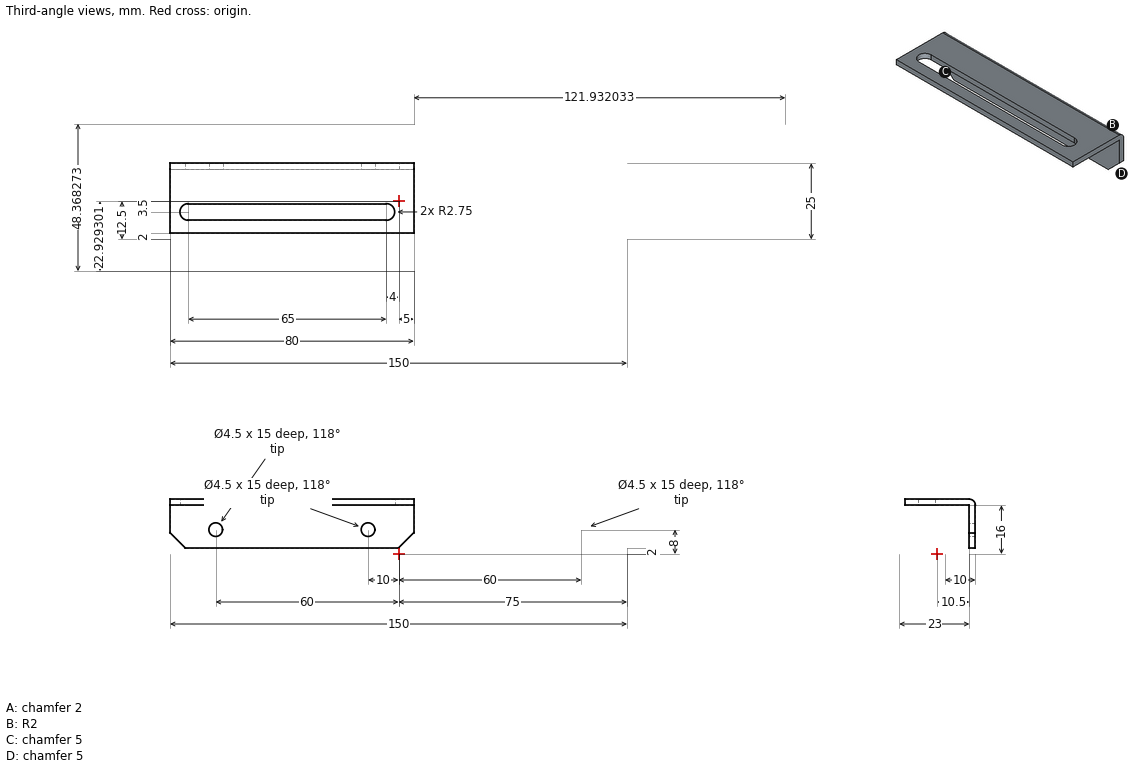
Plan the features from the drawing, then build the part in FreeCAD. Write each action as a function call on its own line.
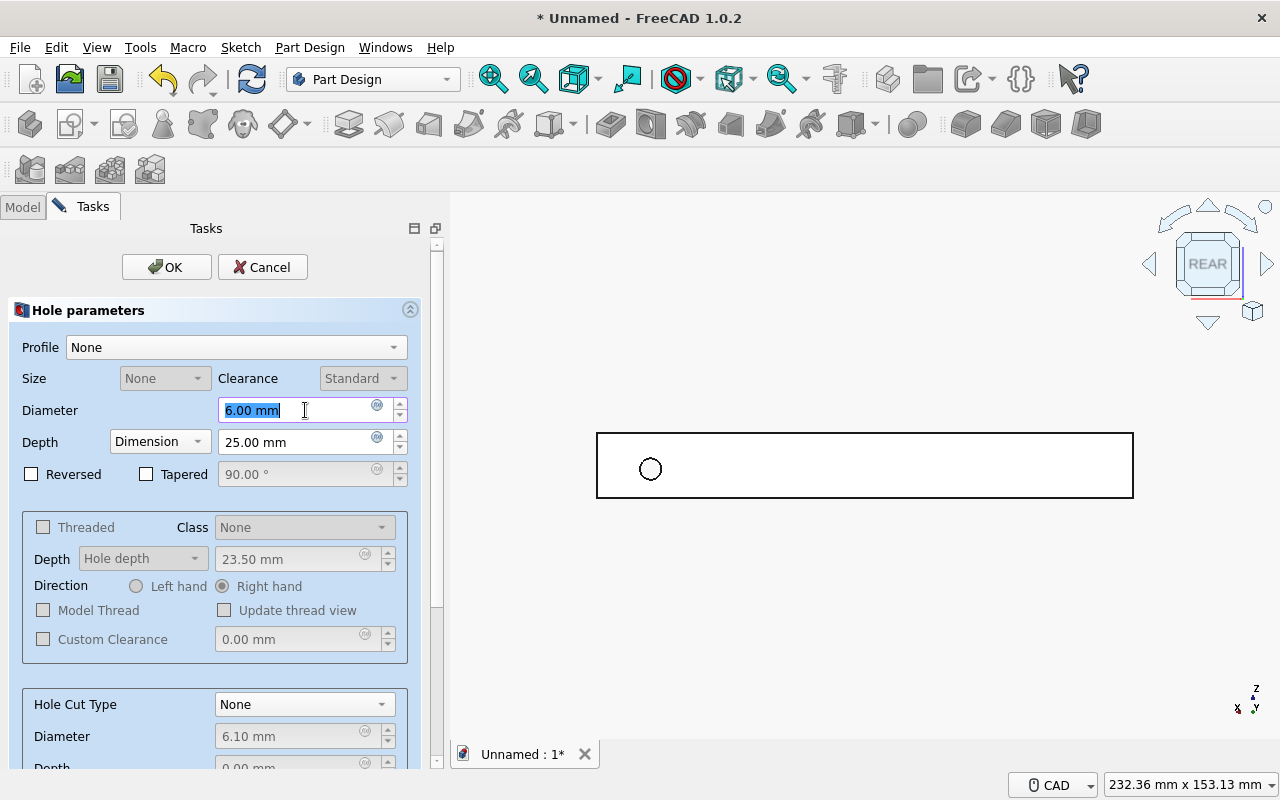
text(4.5)
key(Tab)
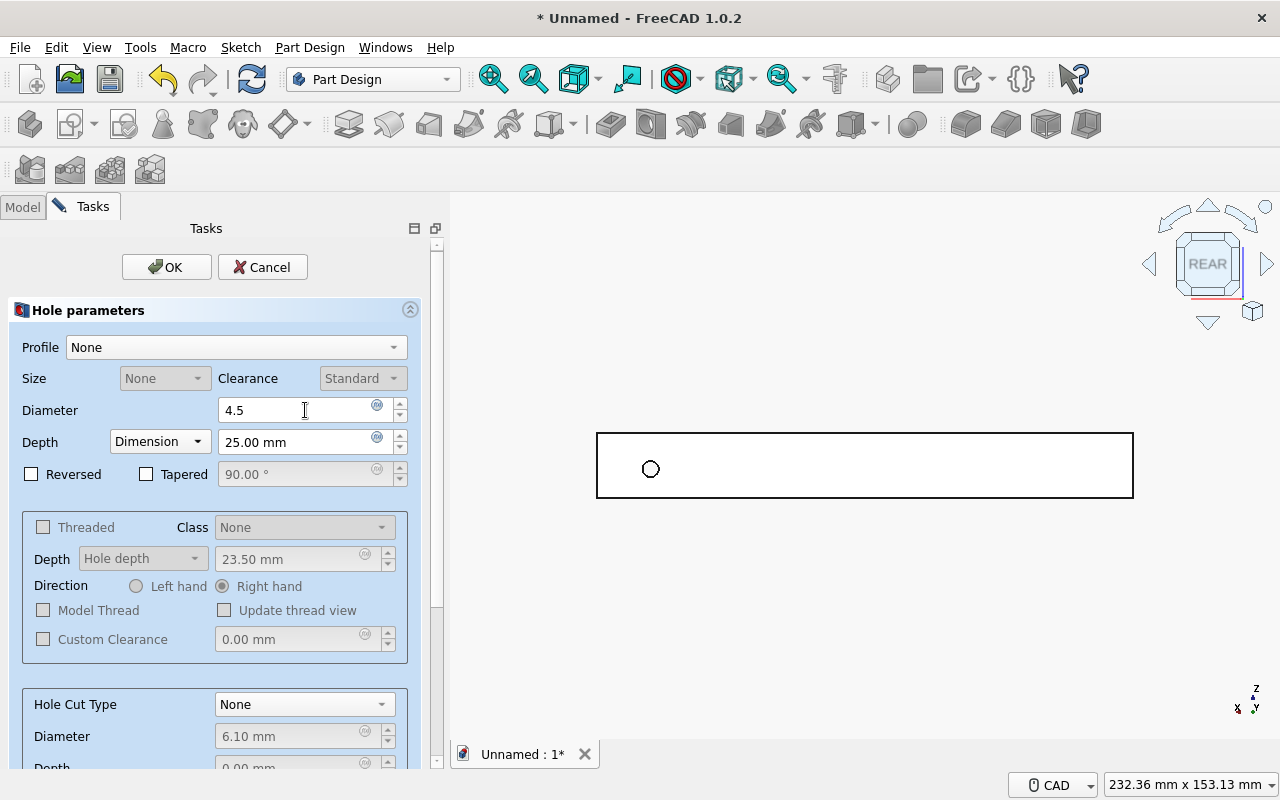
triple_click(305, 442)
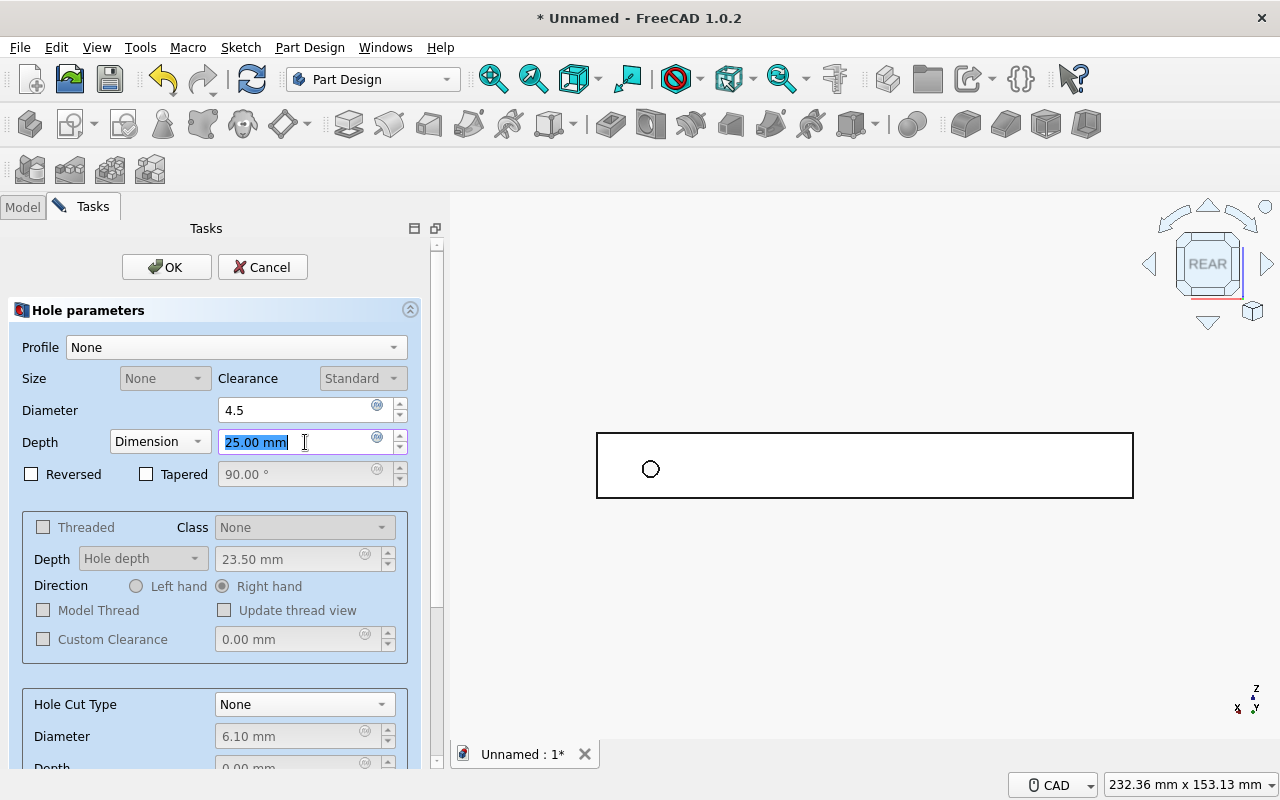
text(15)
key(Tab)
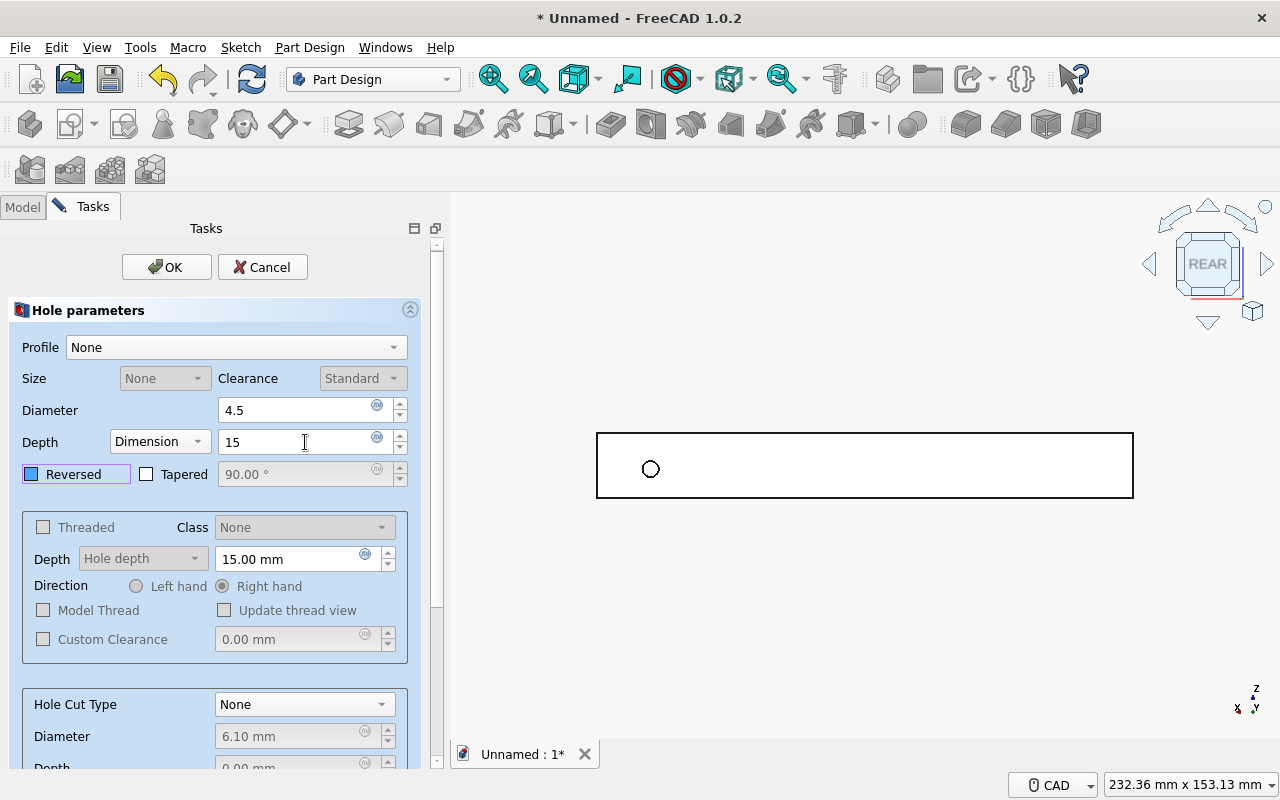
click(167, 267)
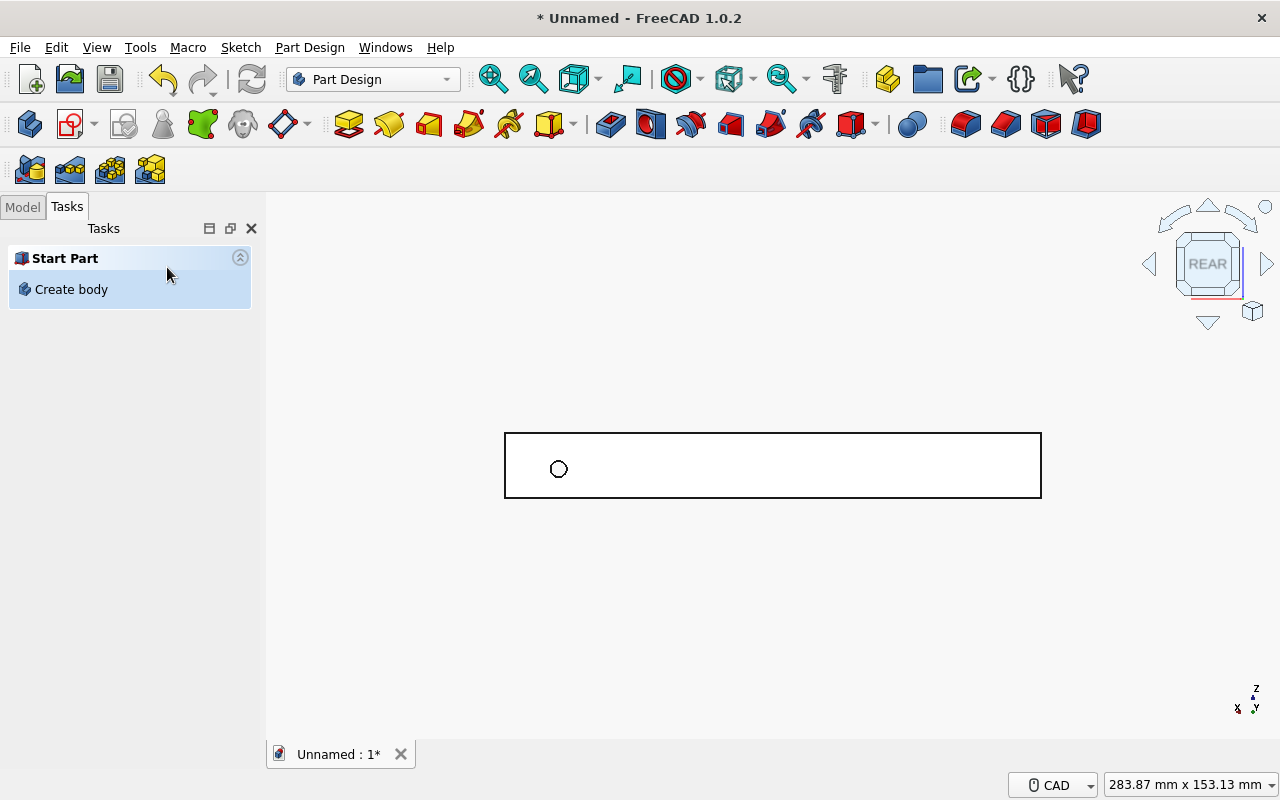
click(620, 464)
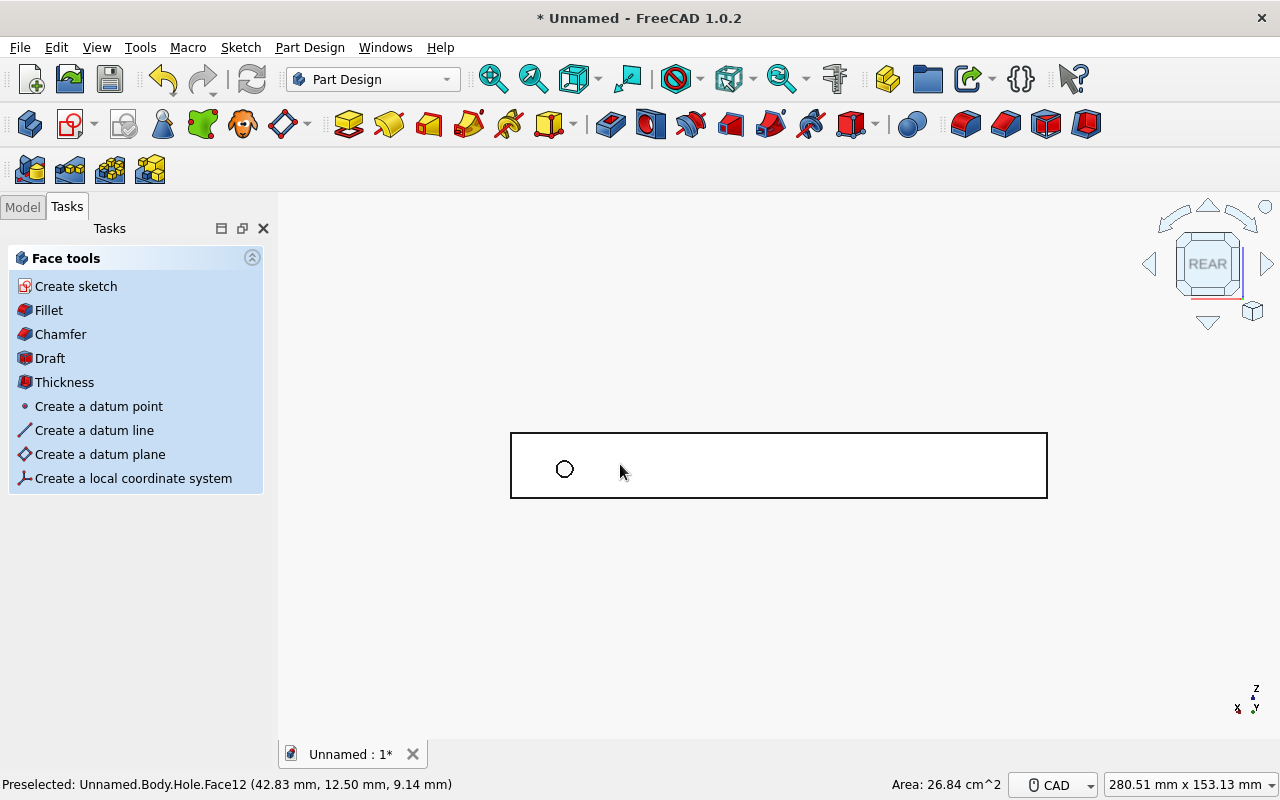
click(70, 124)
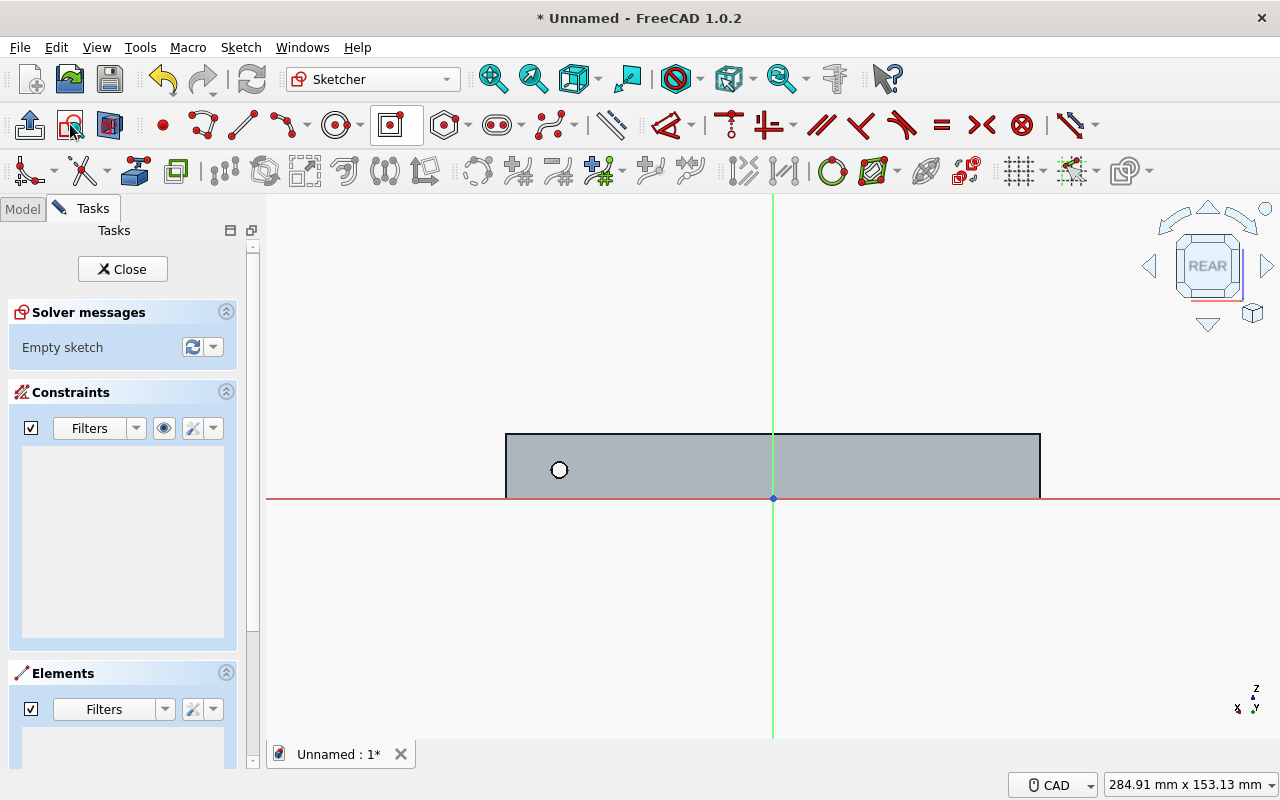
scroll(1001, 470, up, 15)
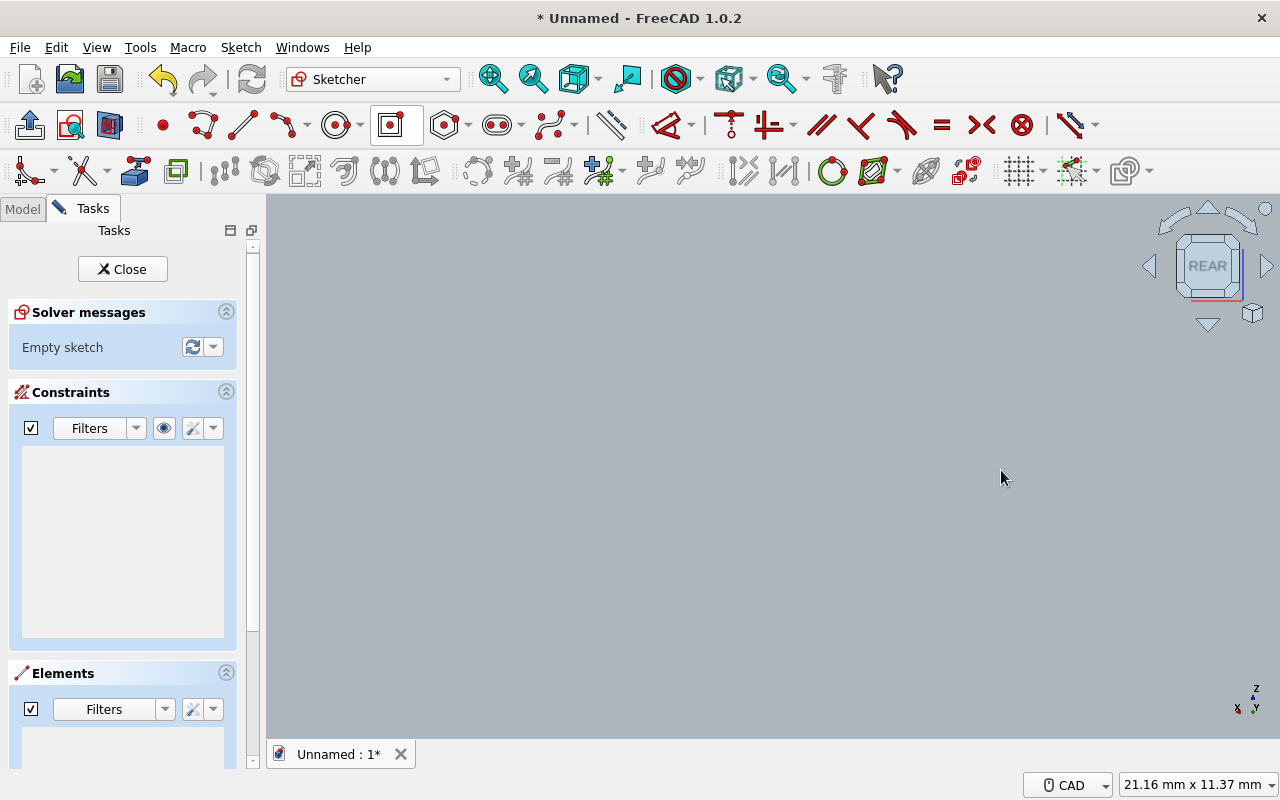
click(336, 126)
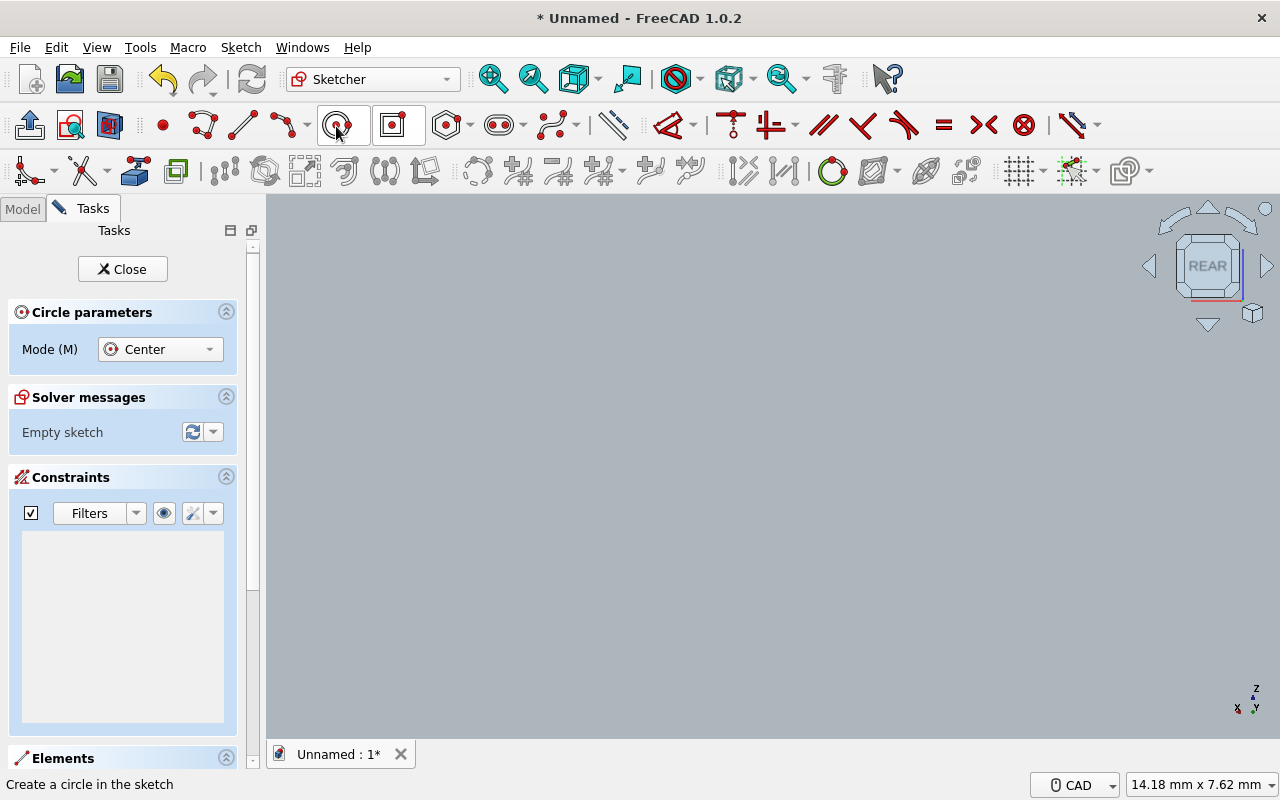
click(697, 462)
click(811, 348)
key(Escape)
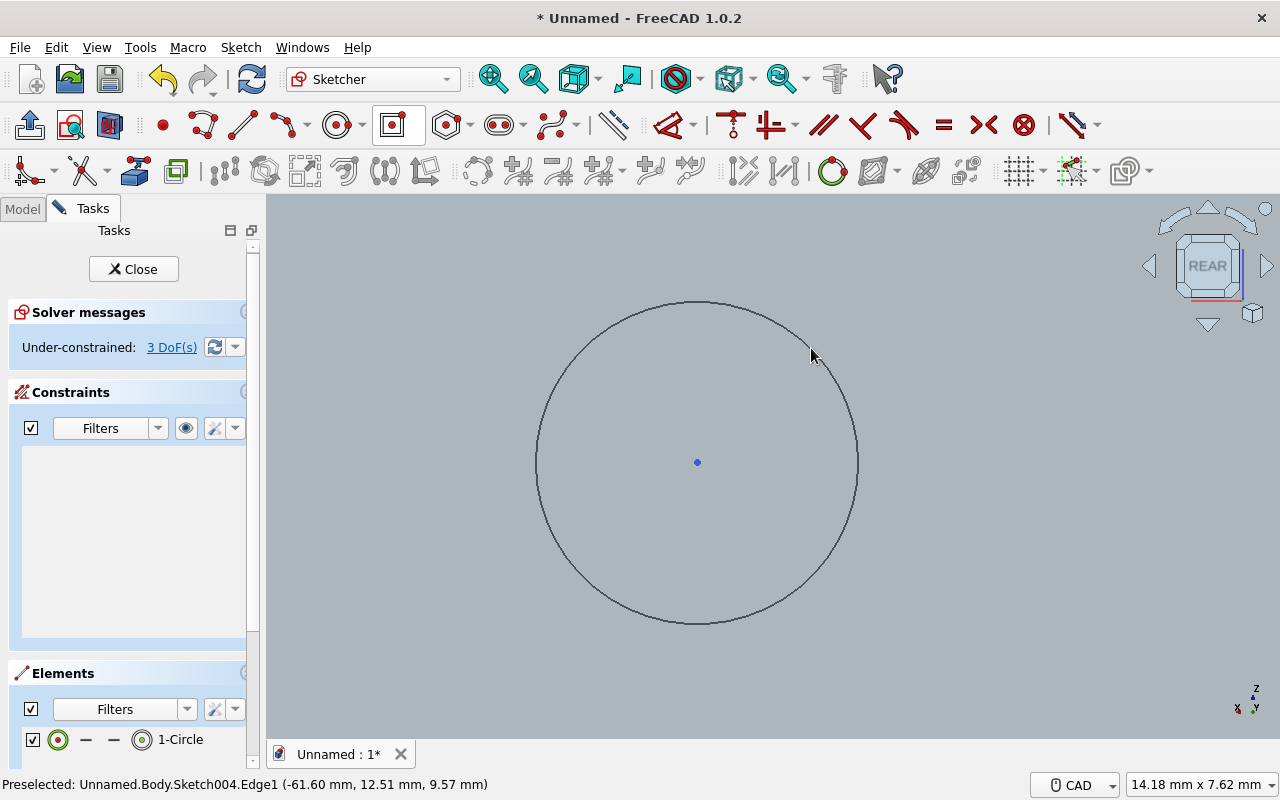
click(668, 126)